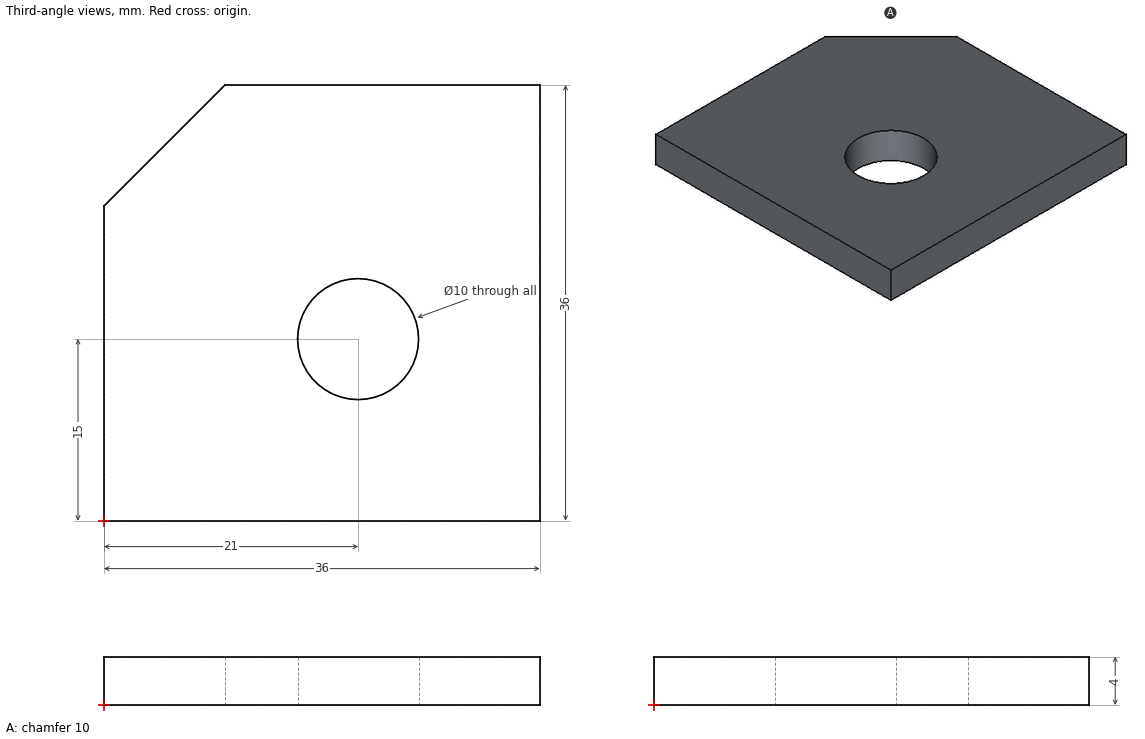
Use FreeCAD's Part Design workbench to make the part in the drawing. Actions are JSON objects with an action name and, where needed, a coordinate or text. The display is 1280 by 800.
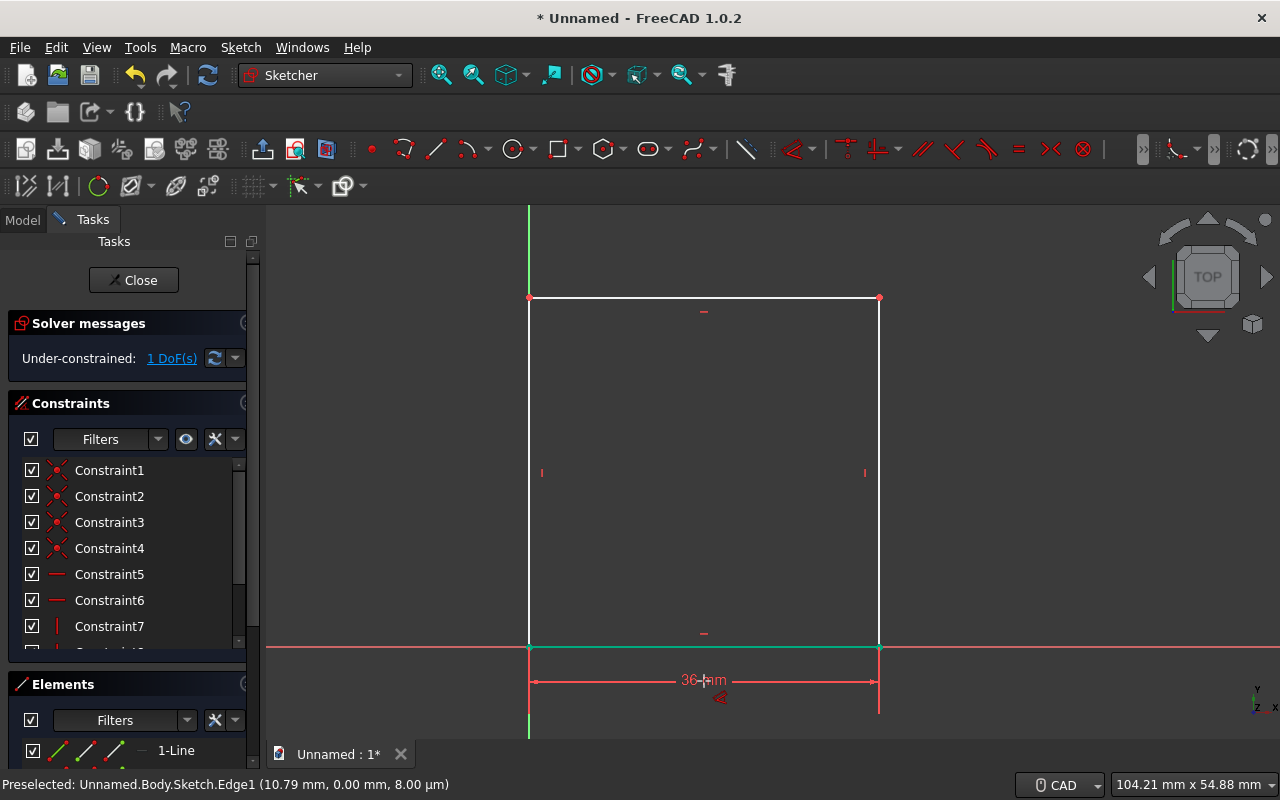
{"action": "left_click", "coordinate": [879, 542]}
{"action": "left_click", "coordinate": [913, 473]}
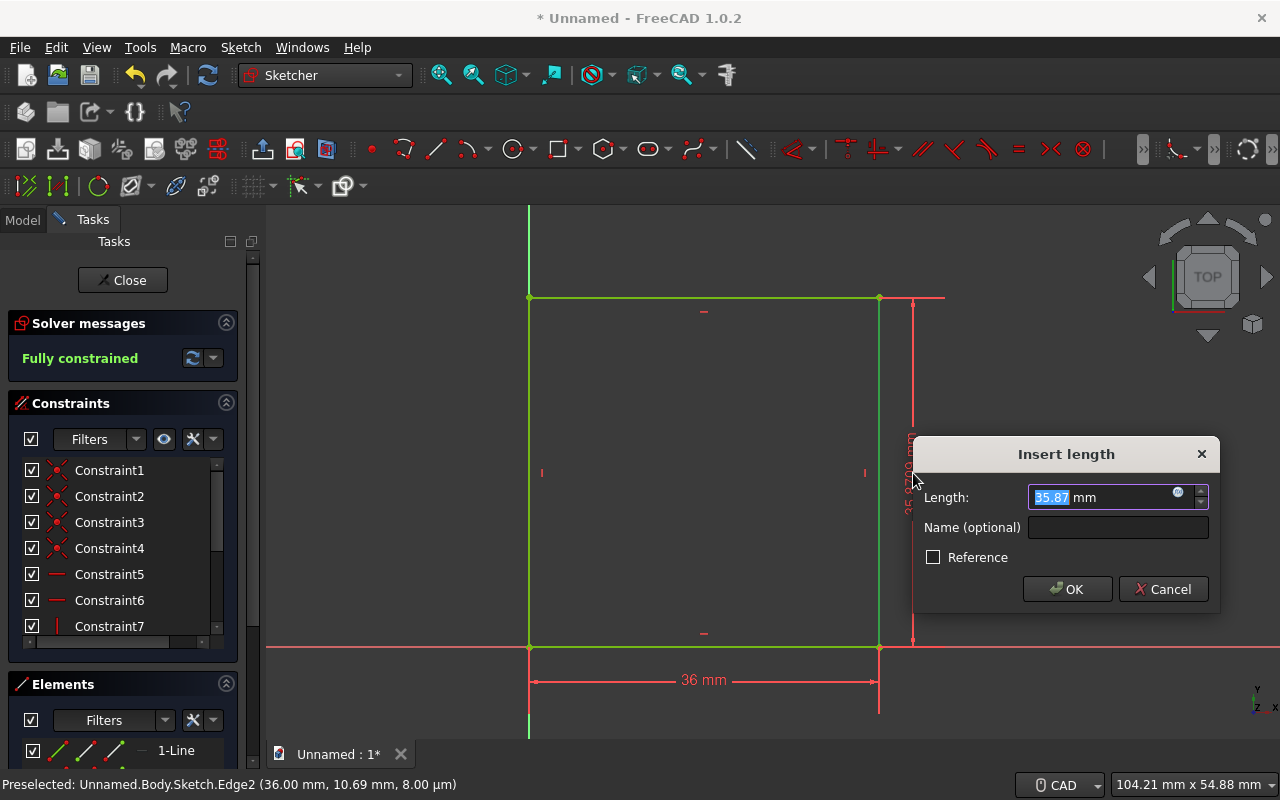
{"action": "type", "text": "36"}
{"action": "key", "text": "Return"}
{"action": "key", "text": "Escape"}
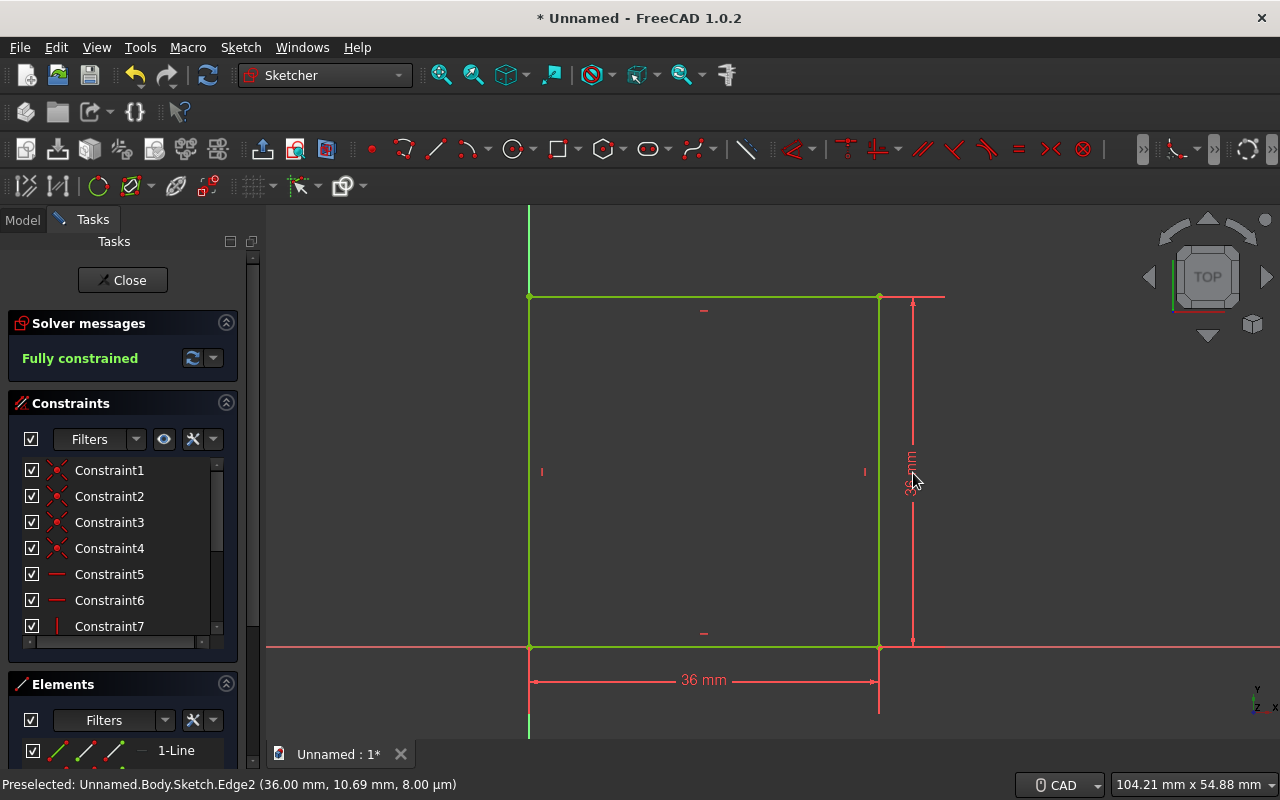
{"action": "left_click", "coordinate": [123, 280]}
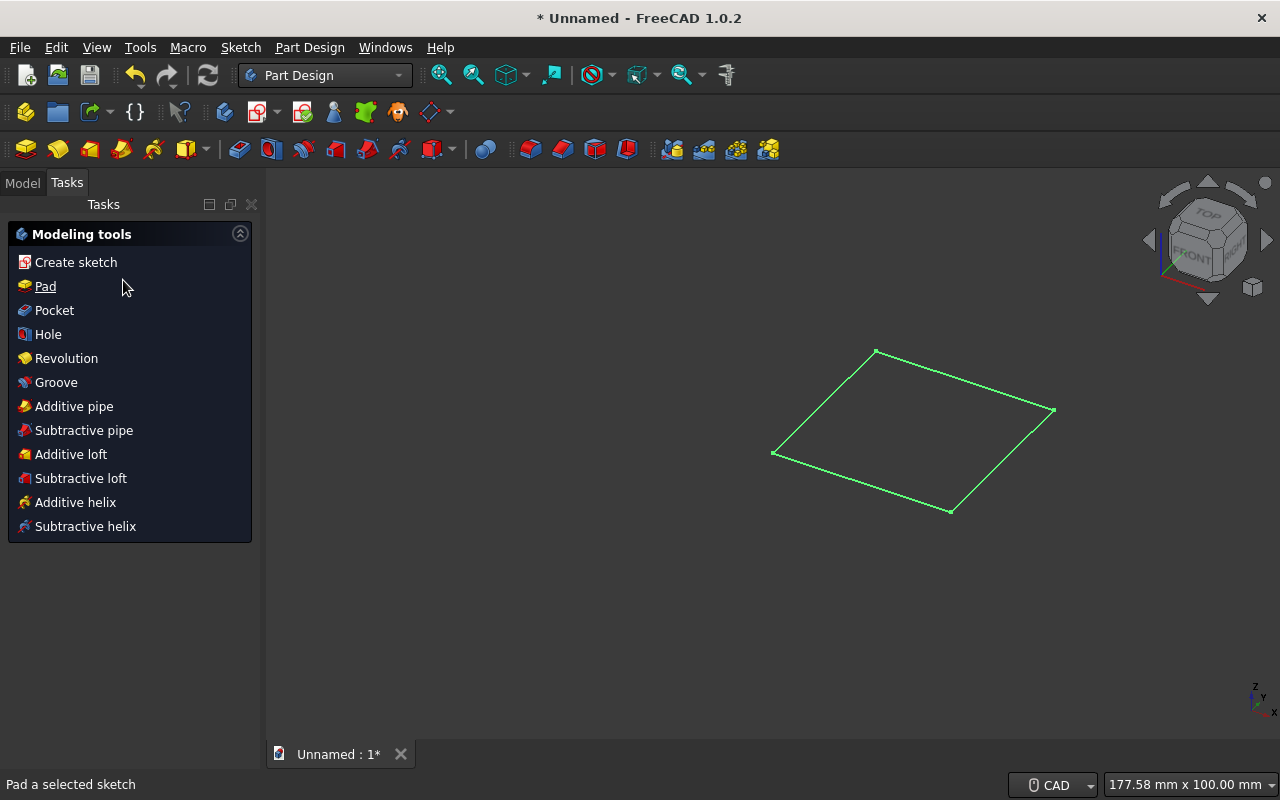
{"action": "left_click", "coordinate": [26, 150]}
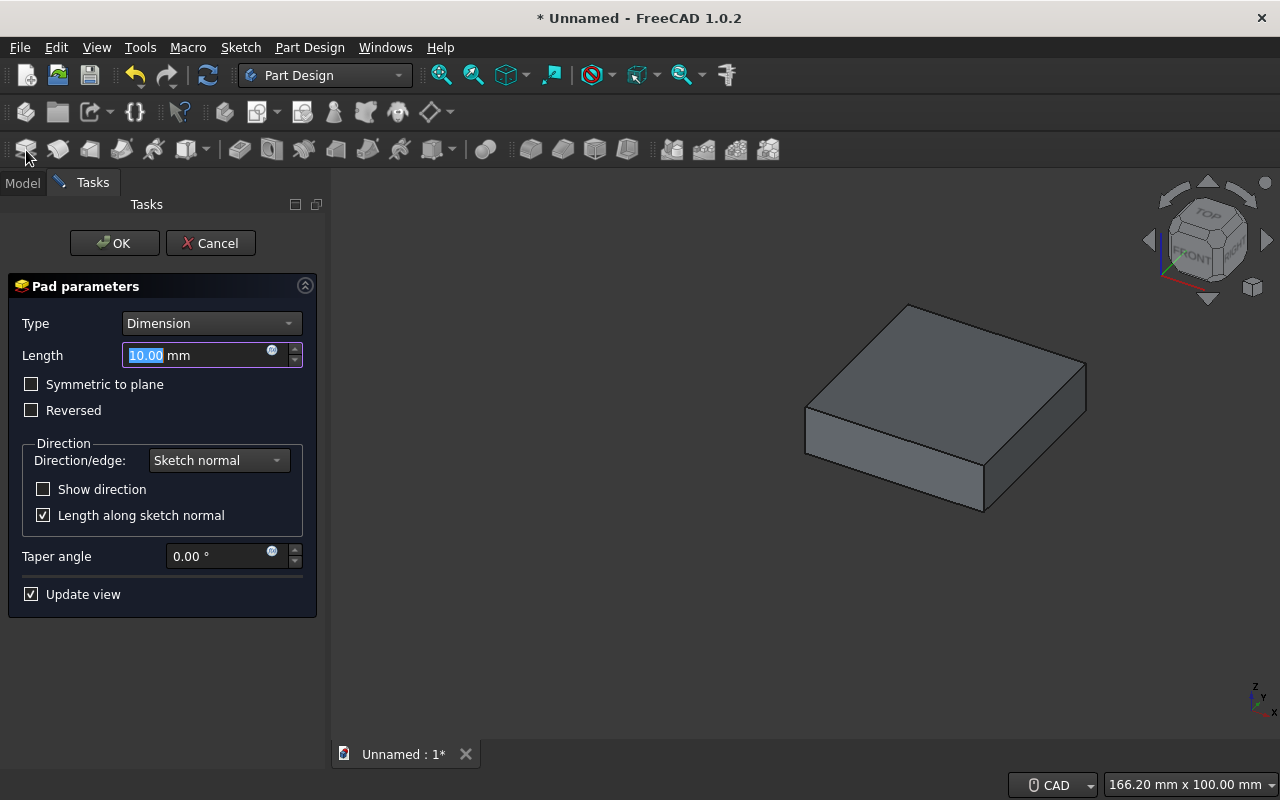
{"action": "type", "text": "4"}
{"action": "key", "text": "Tab"}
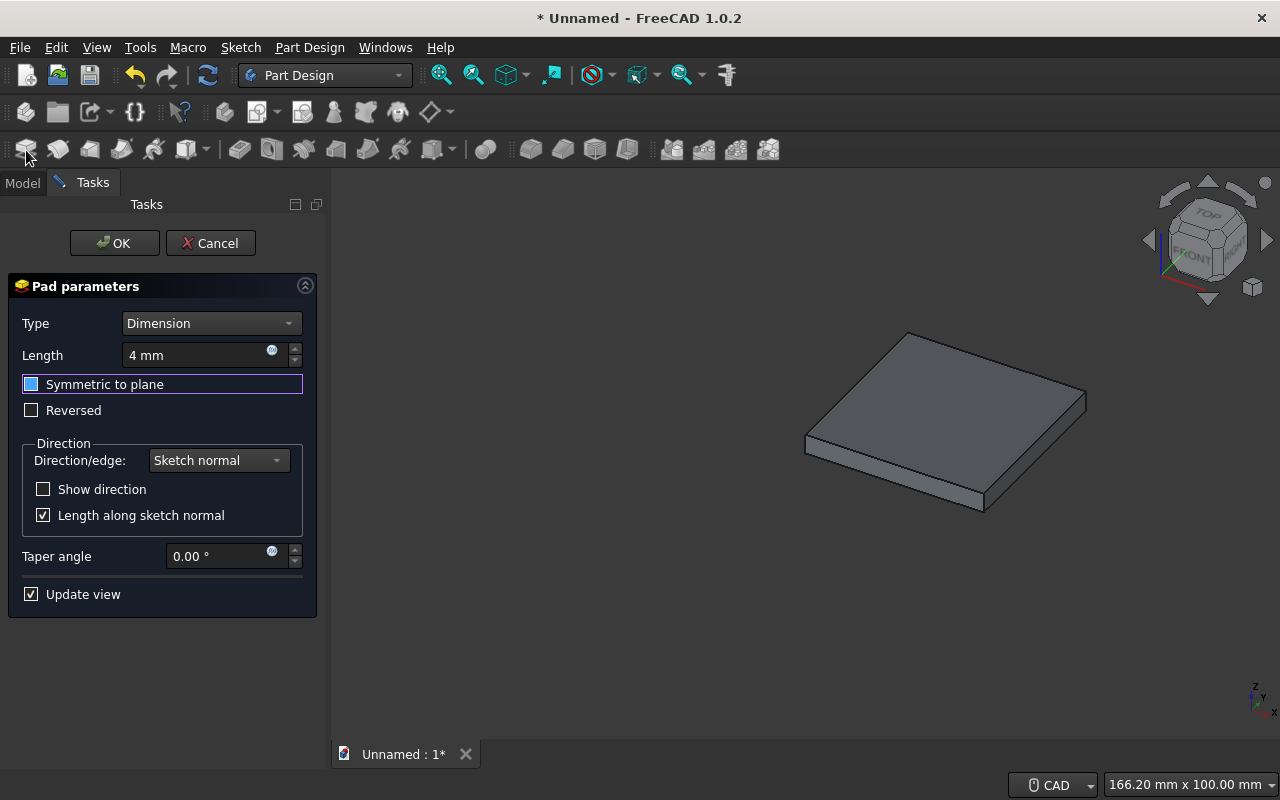
{"action": "left_click", "coordinate": [115, 243]}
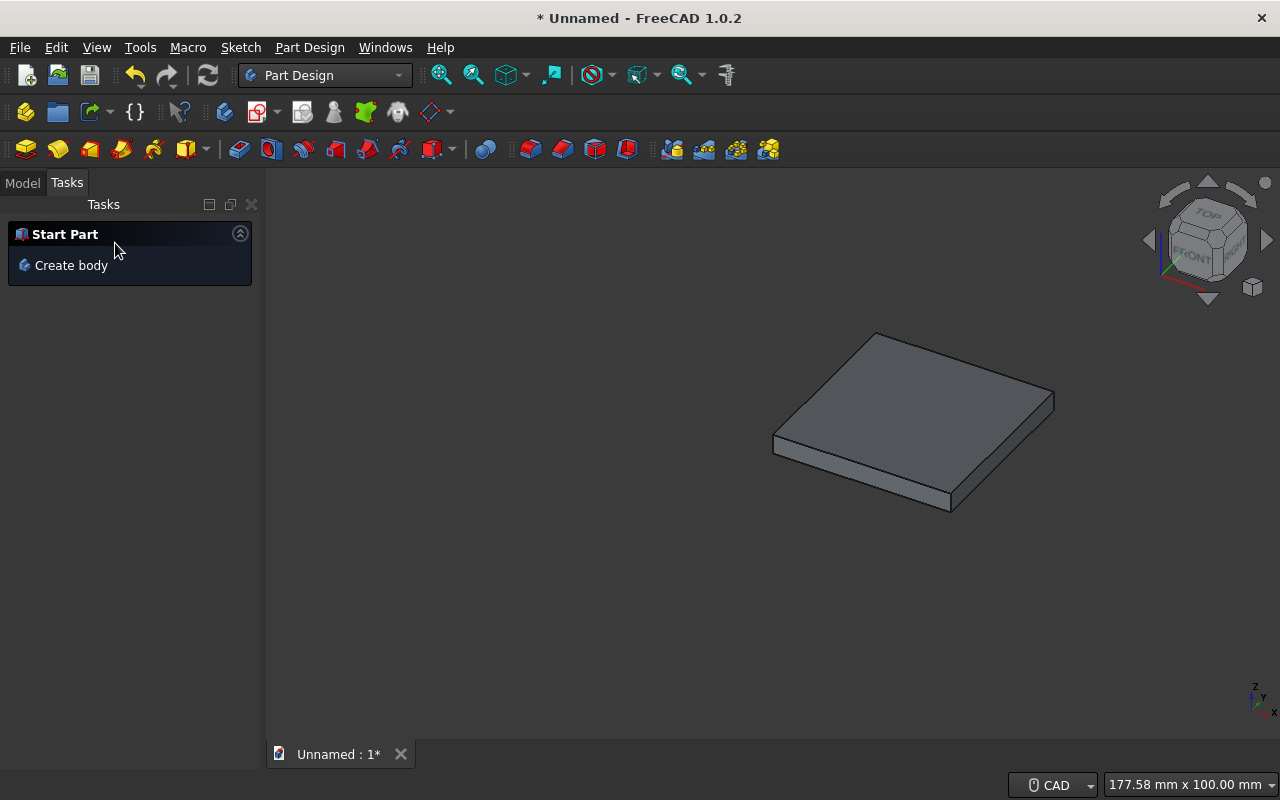
{"action": "key", "text": "v f"}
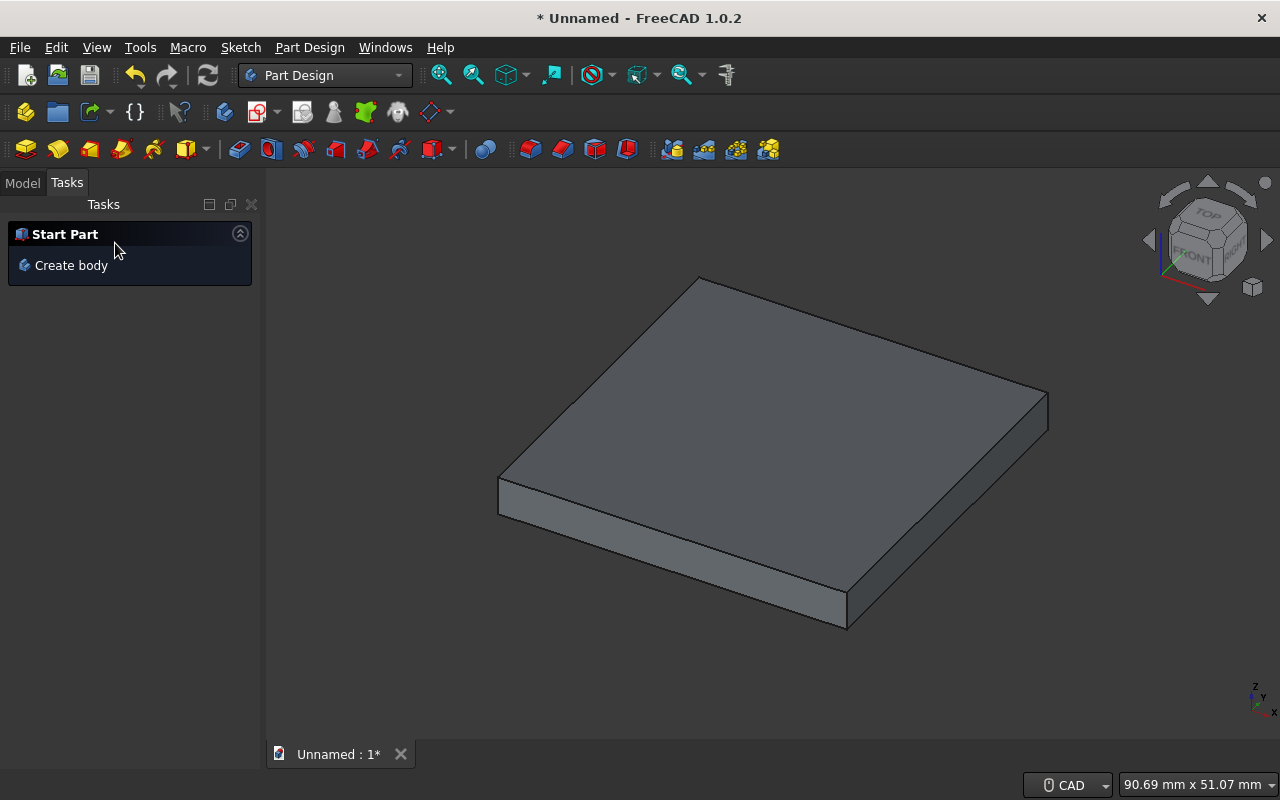
{"action": "key", "text": "0"}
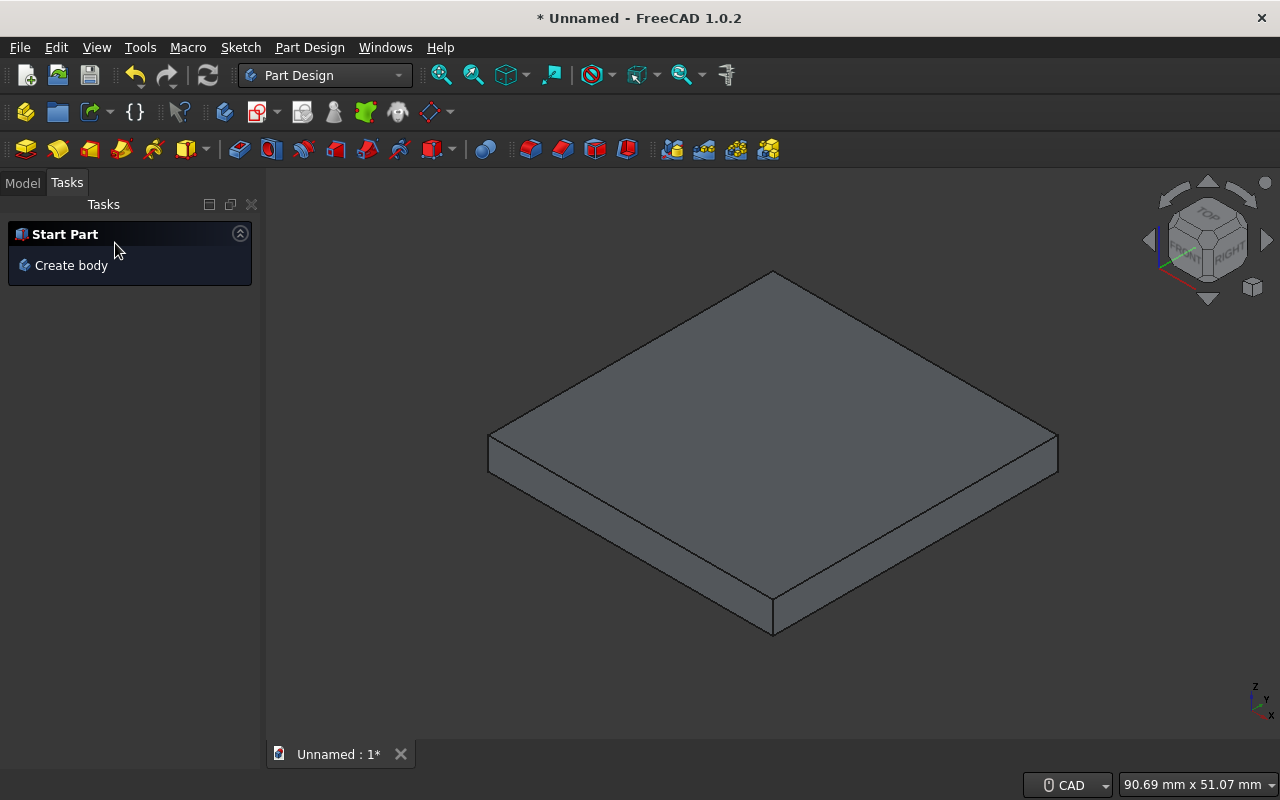
{"action": "key", "text": "2"}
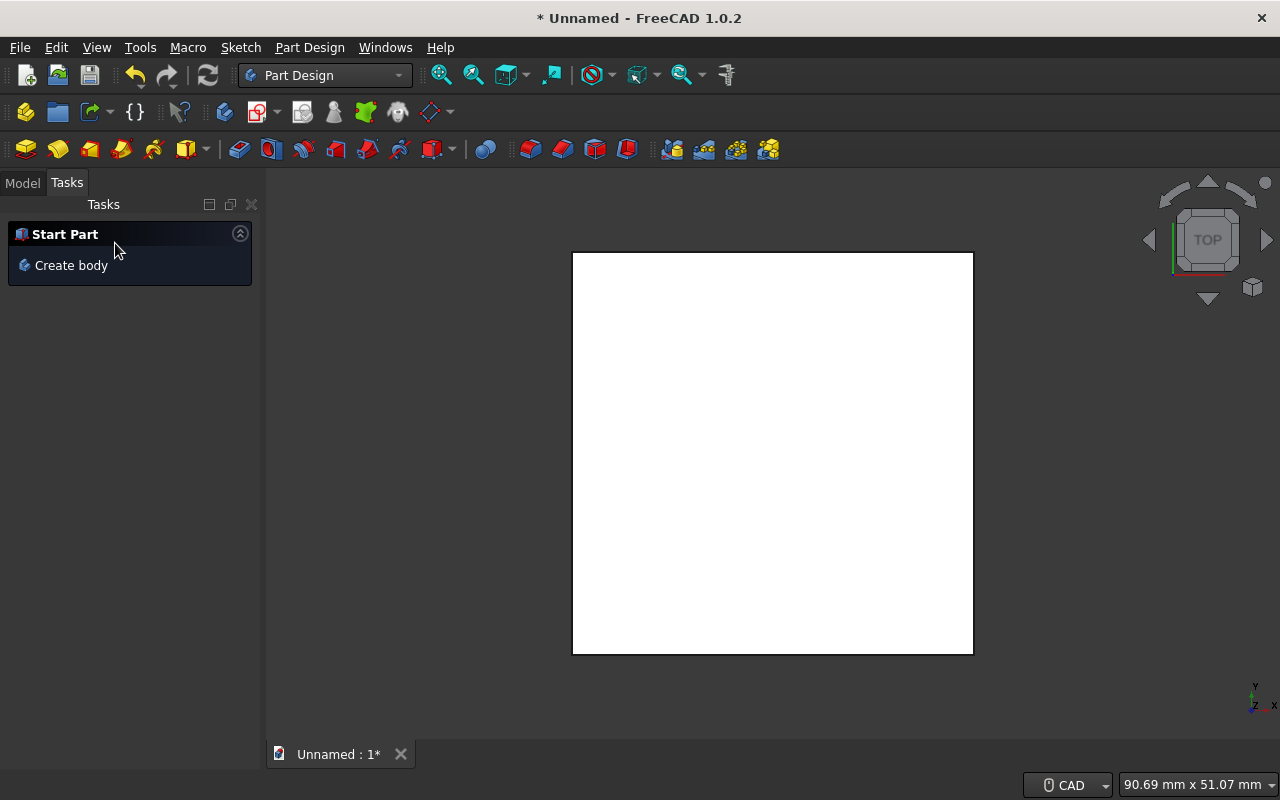
{"action": "key", "text": "1"}